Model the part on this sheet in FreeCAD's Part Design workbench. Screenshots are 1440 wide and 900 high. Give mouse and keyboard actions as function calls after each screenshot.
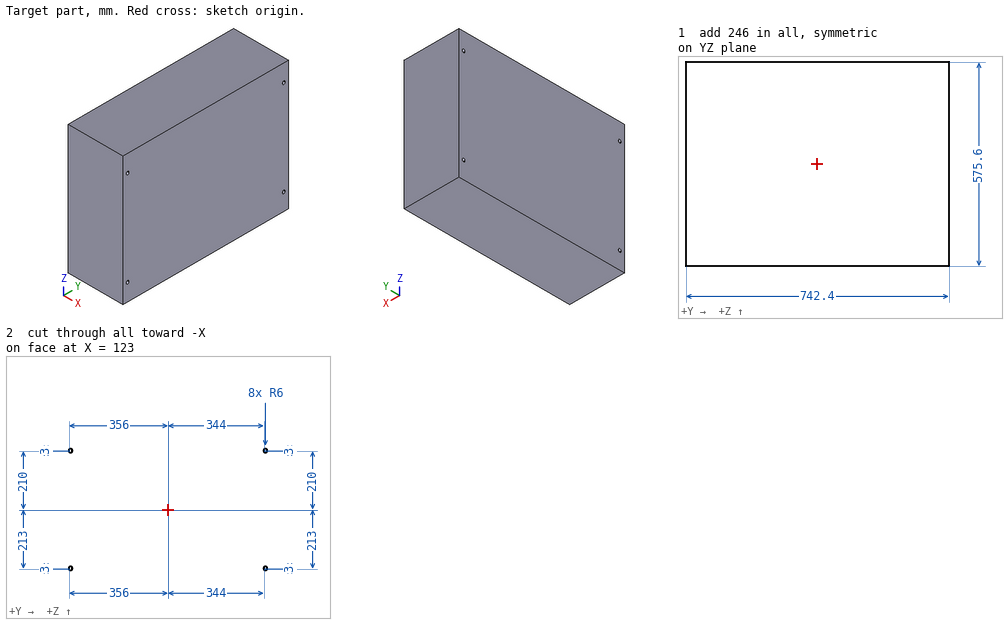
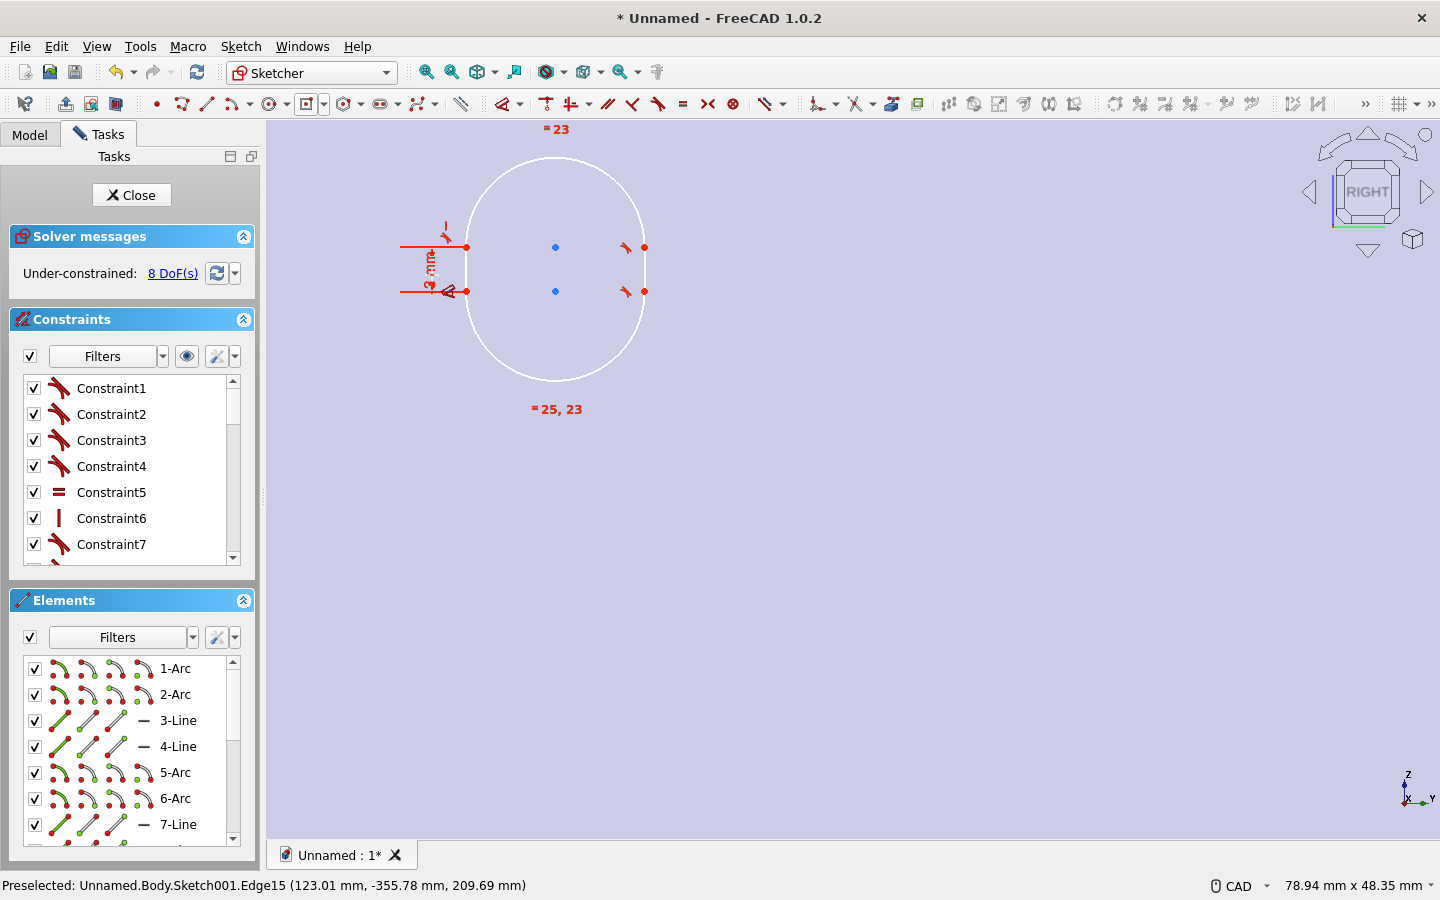
scroll(463, 290, down, 14)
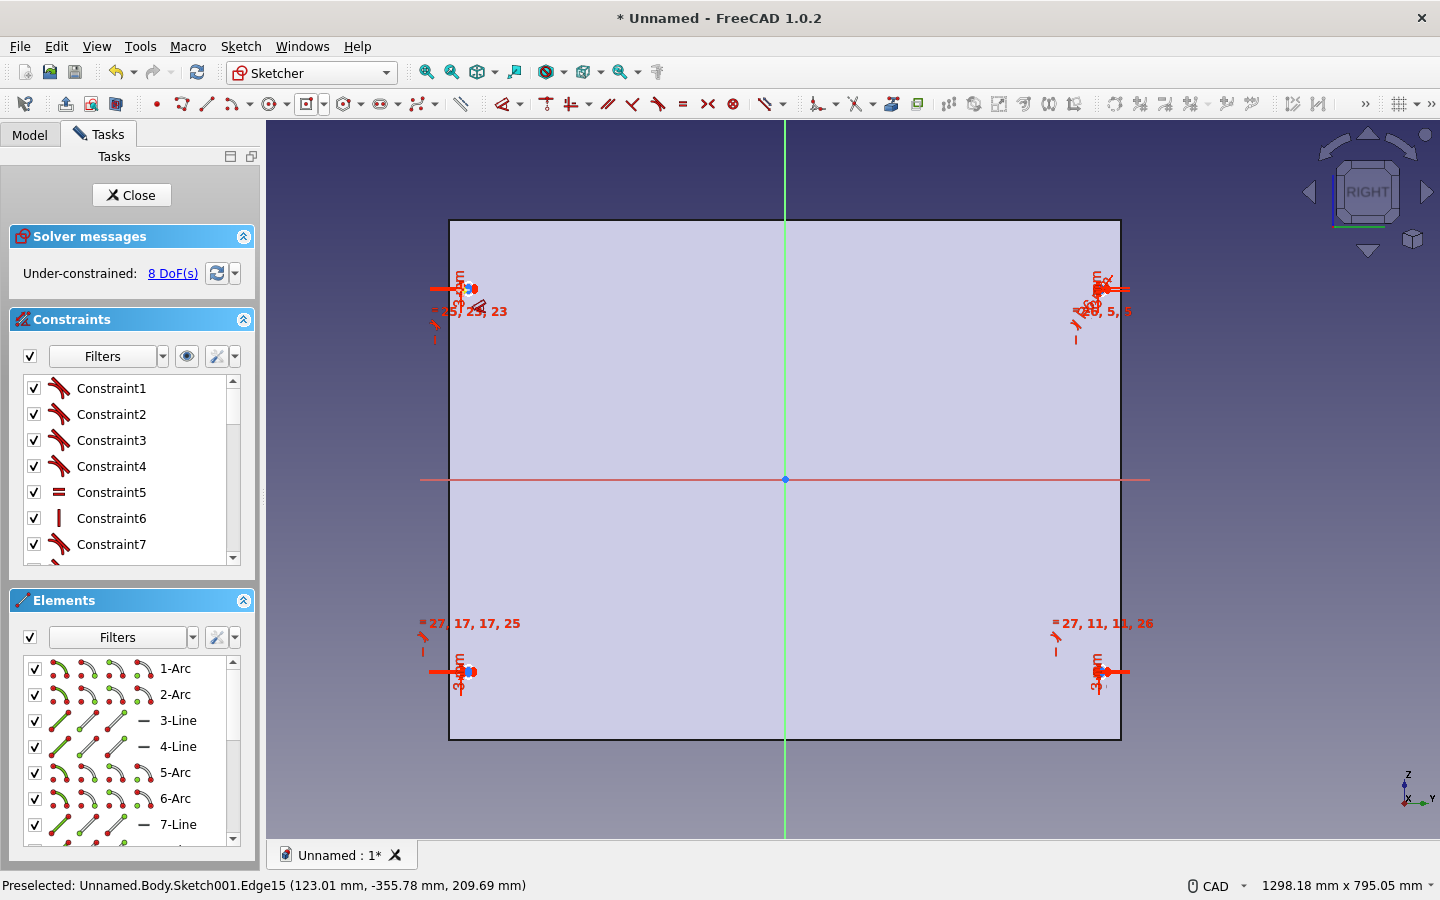
scroll(1096, 291, up, 8)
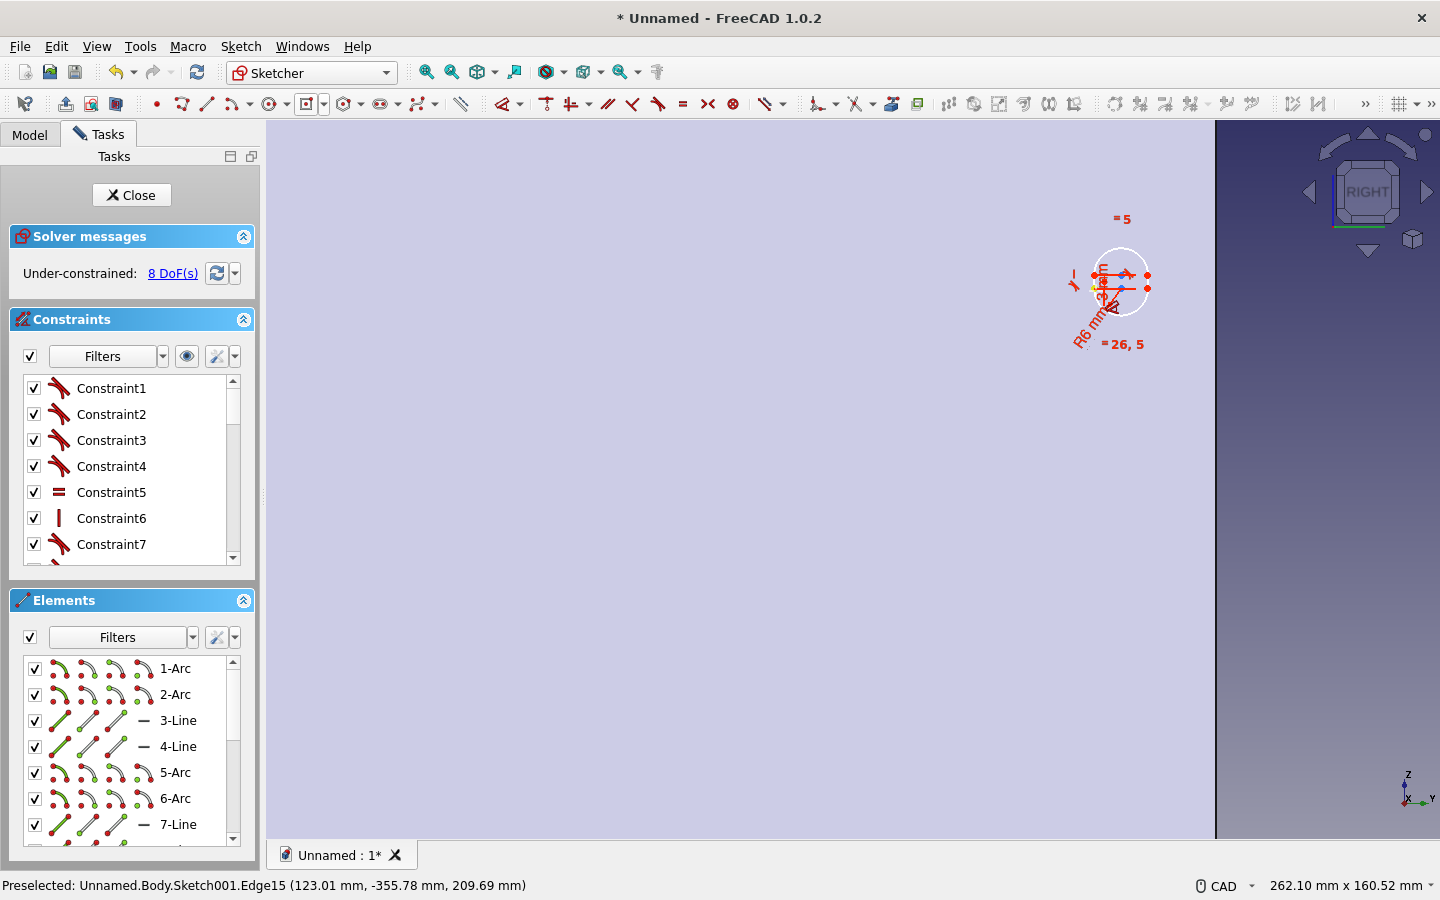
click(1094, 289)
click(694, 255)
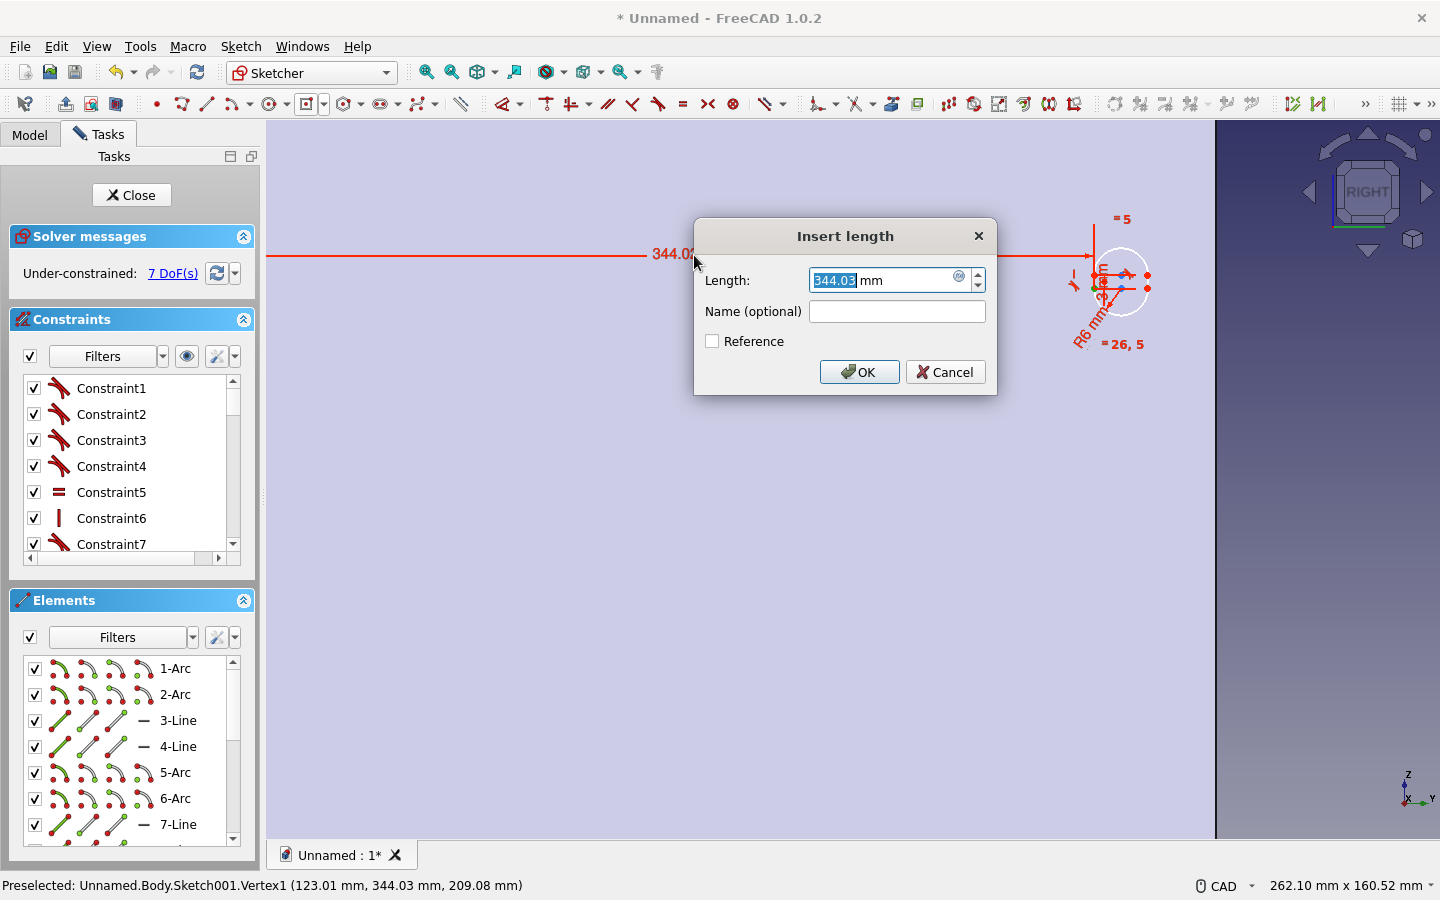
text(344)
key(Return)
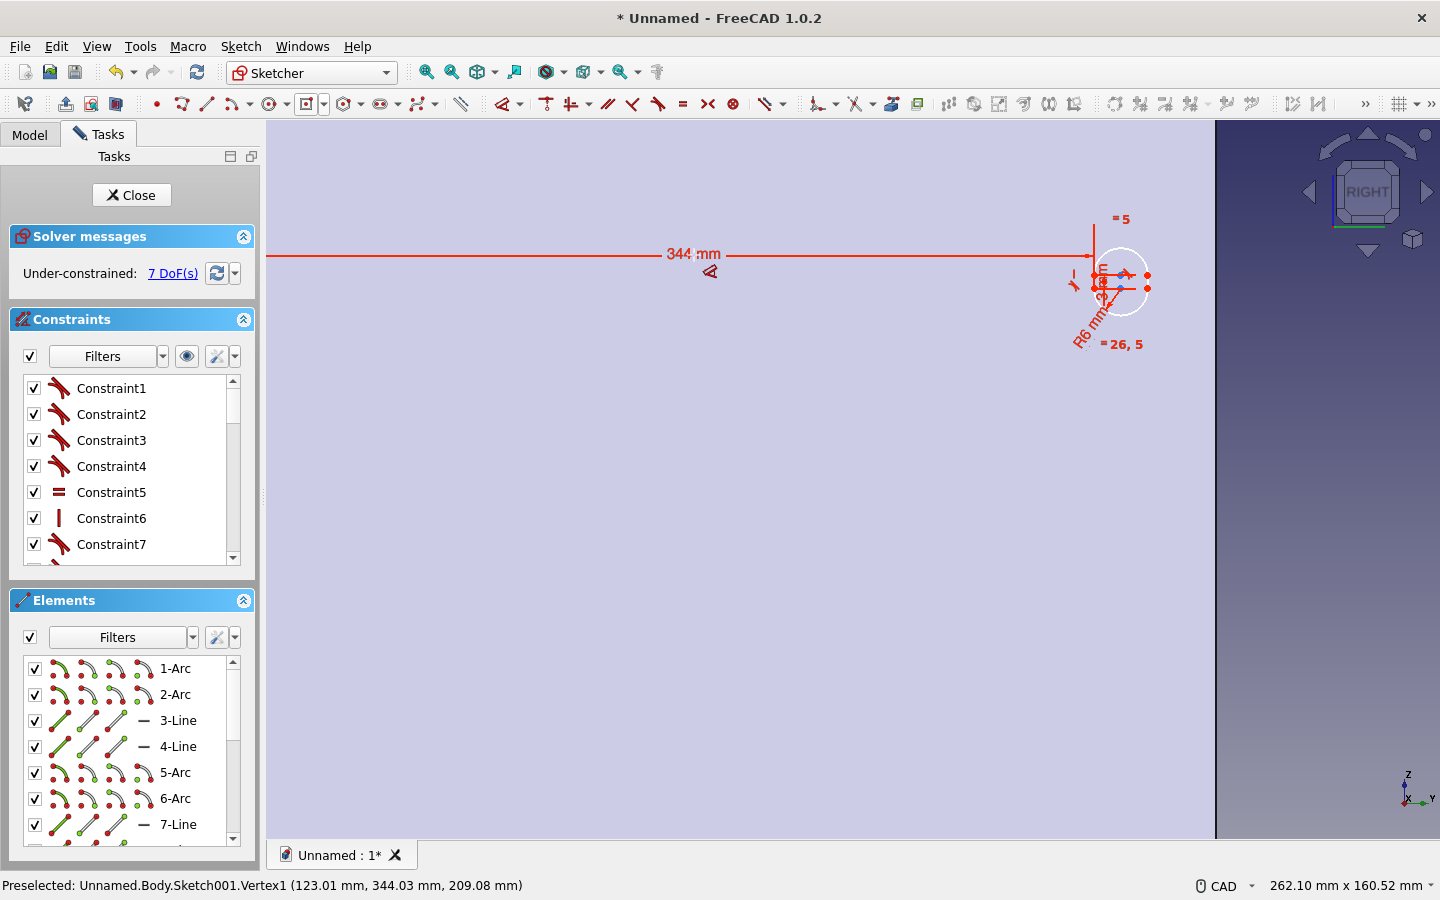
click(1094, 289)
click(1128, 550)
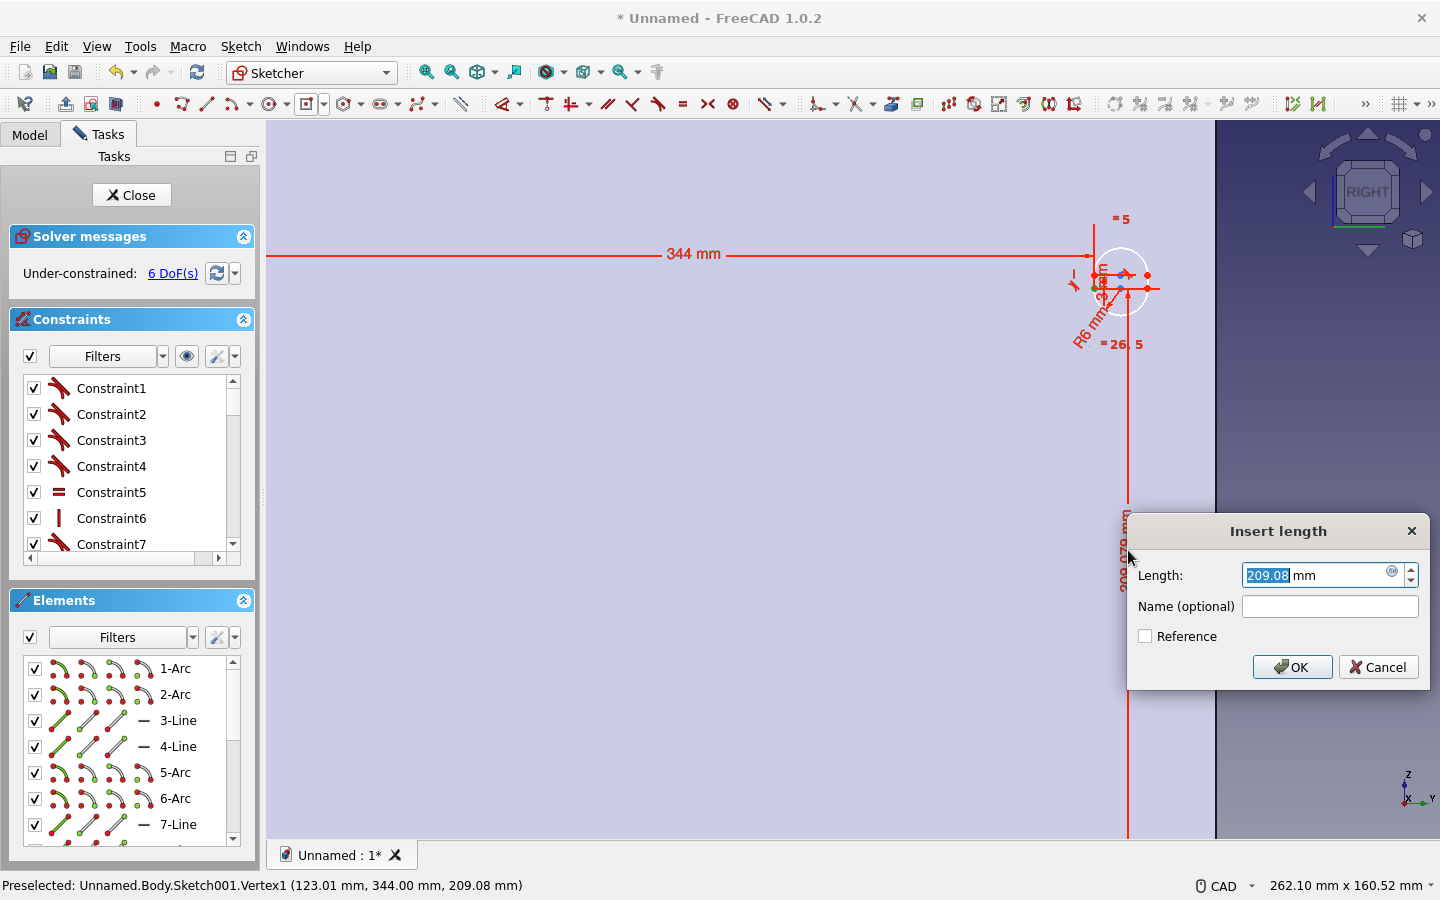
text(210)
key(Return)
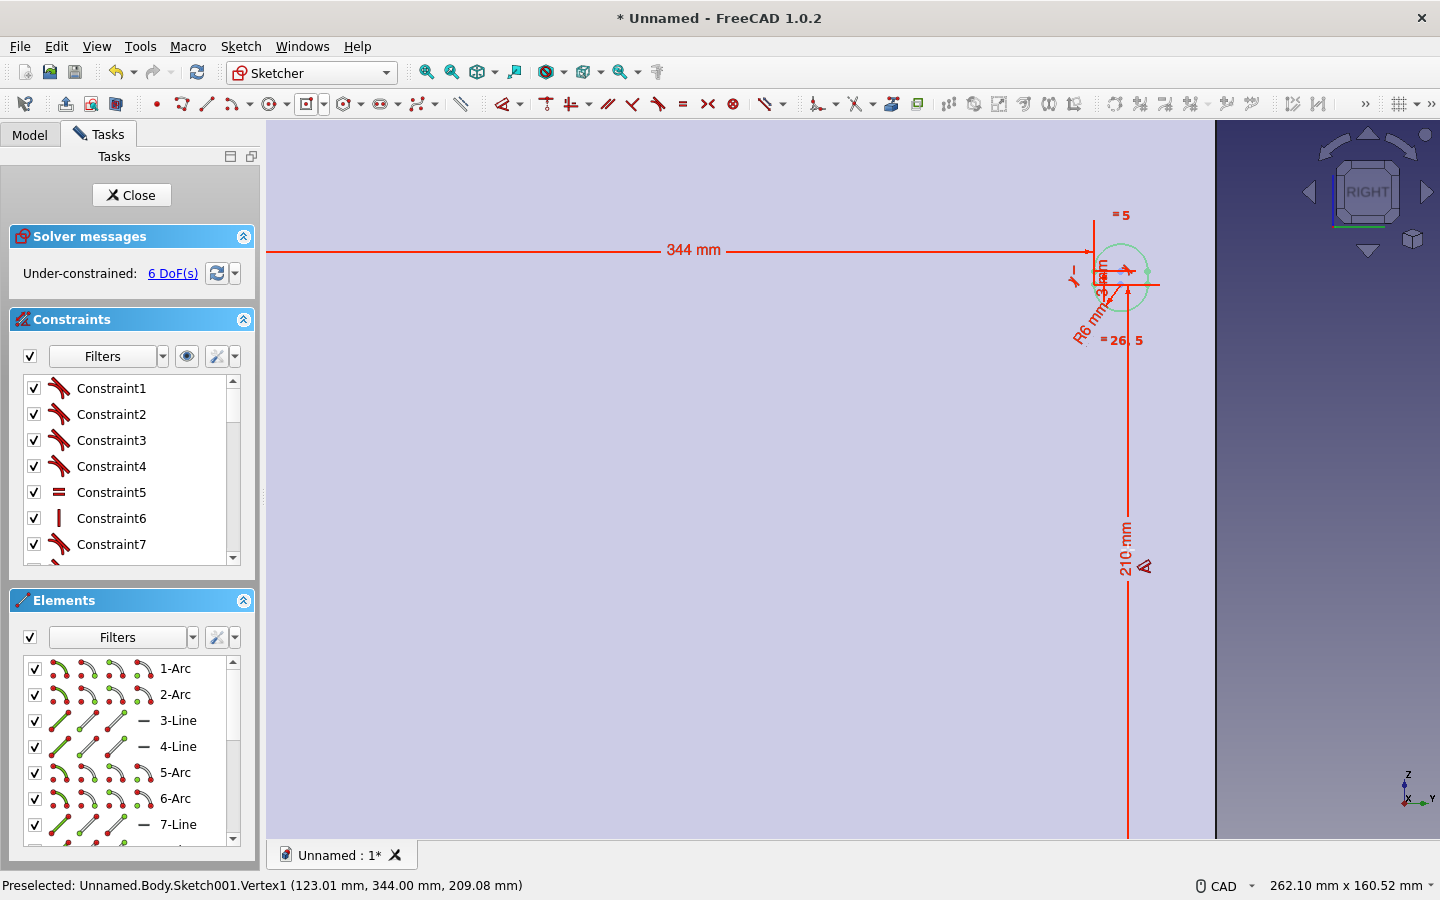
scroll(1096, 291, down, 8)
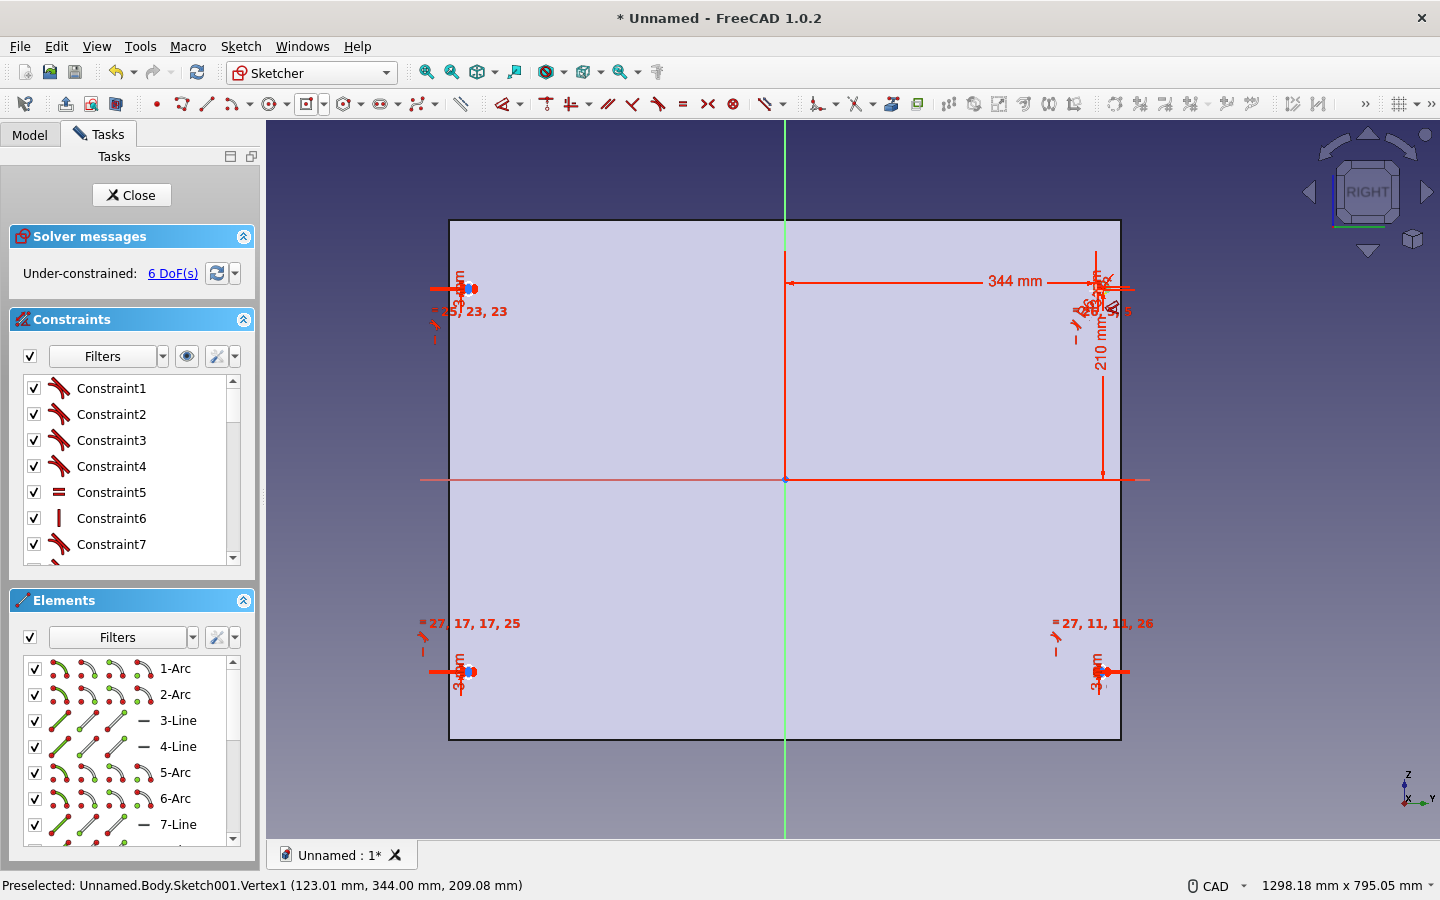
scroll(1096, 673, up, 8)